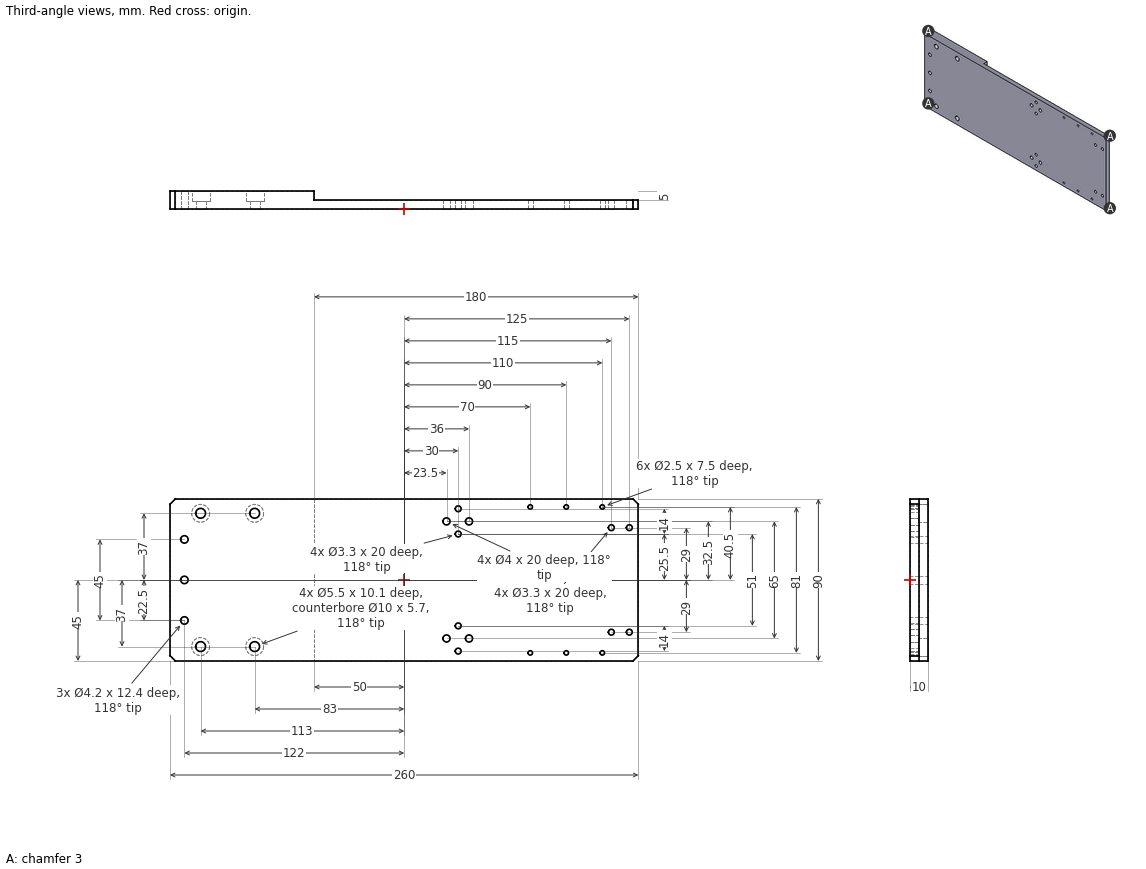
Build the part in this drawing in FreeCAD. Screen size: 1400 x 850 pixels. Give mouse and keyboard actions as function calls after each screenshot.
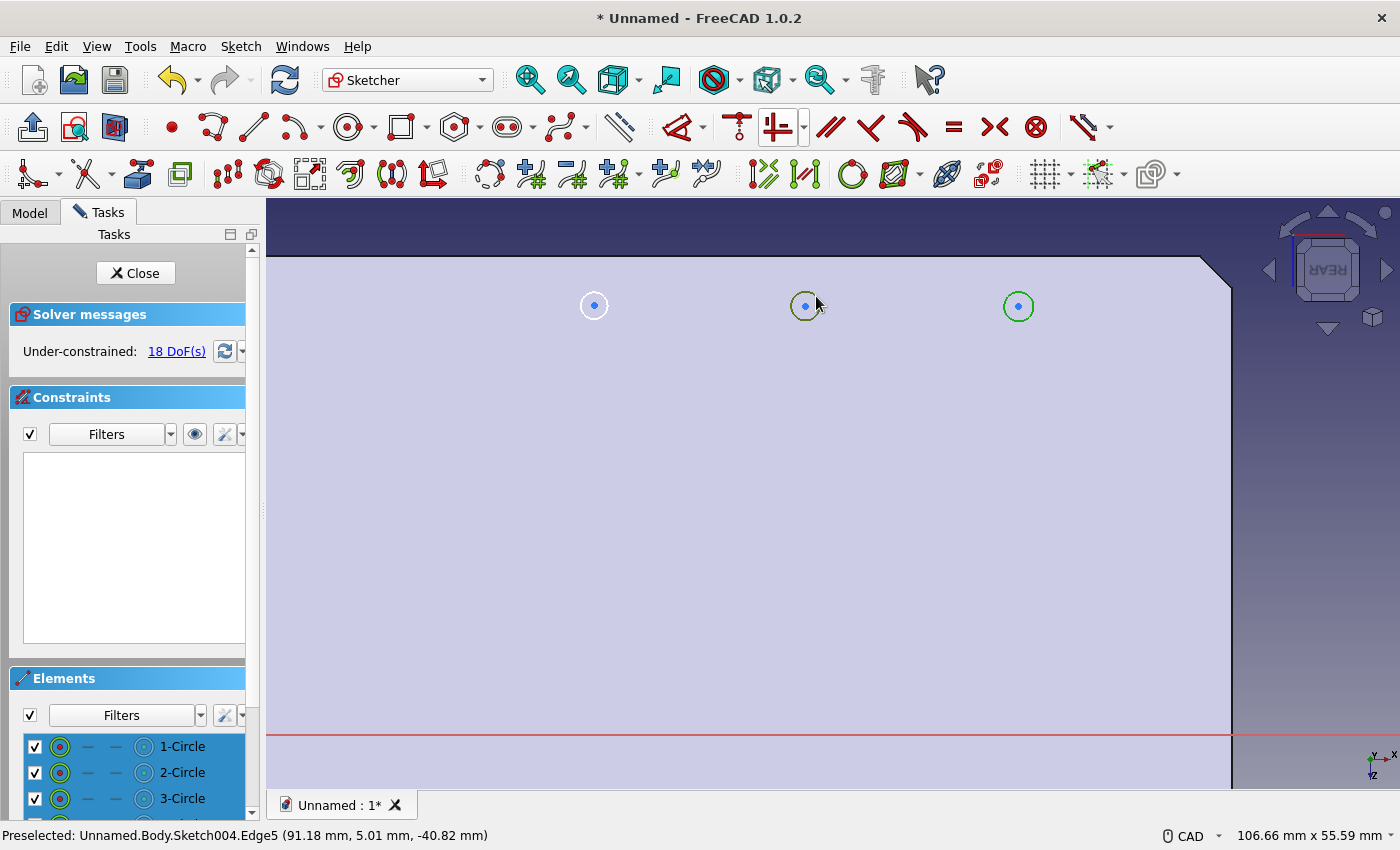
click(604, 296)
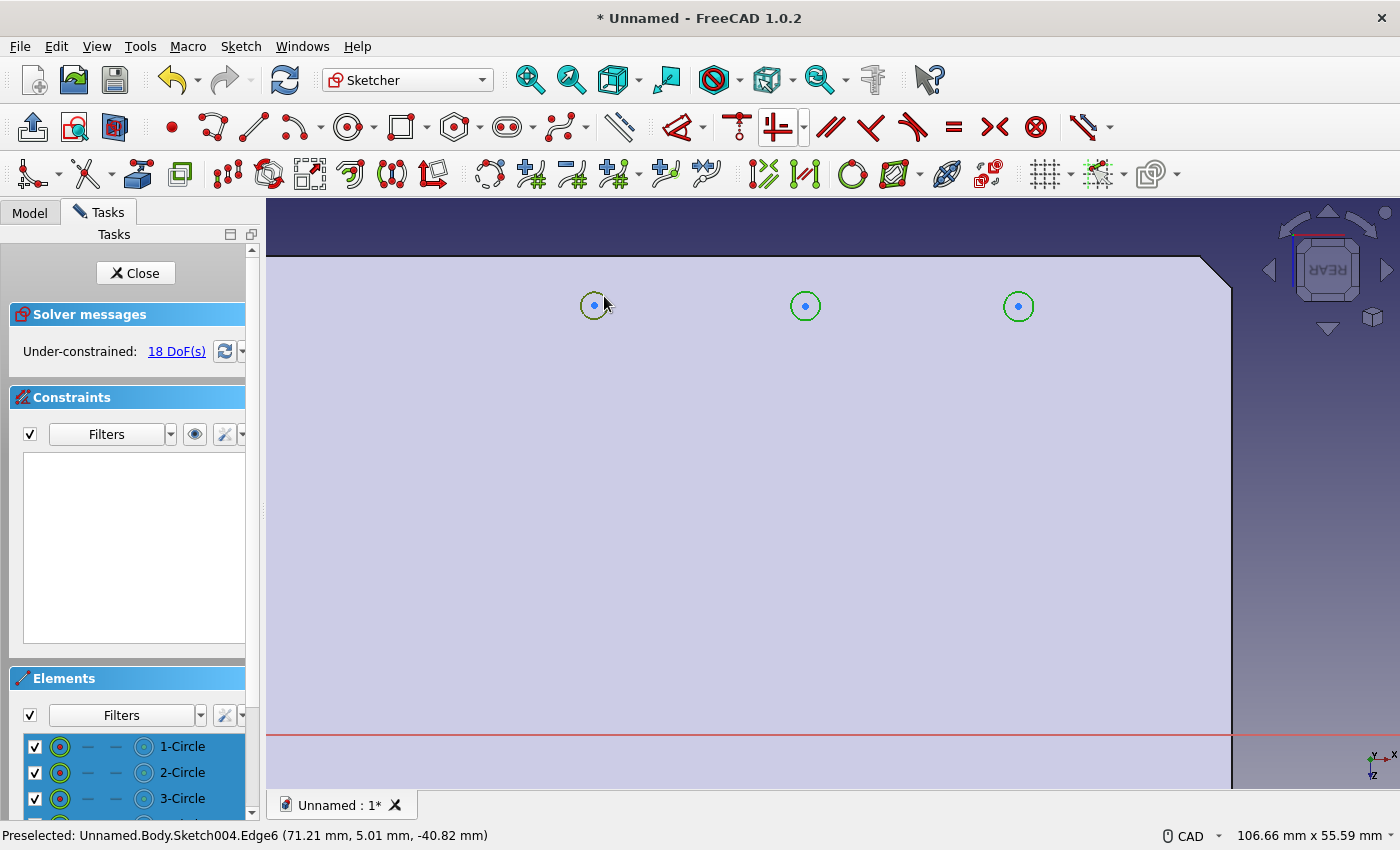
click(954, 128)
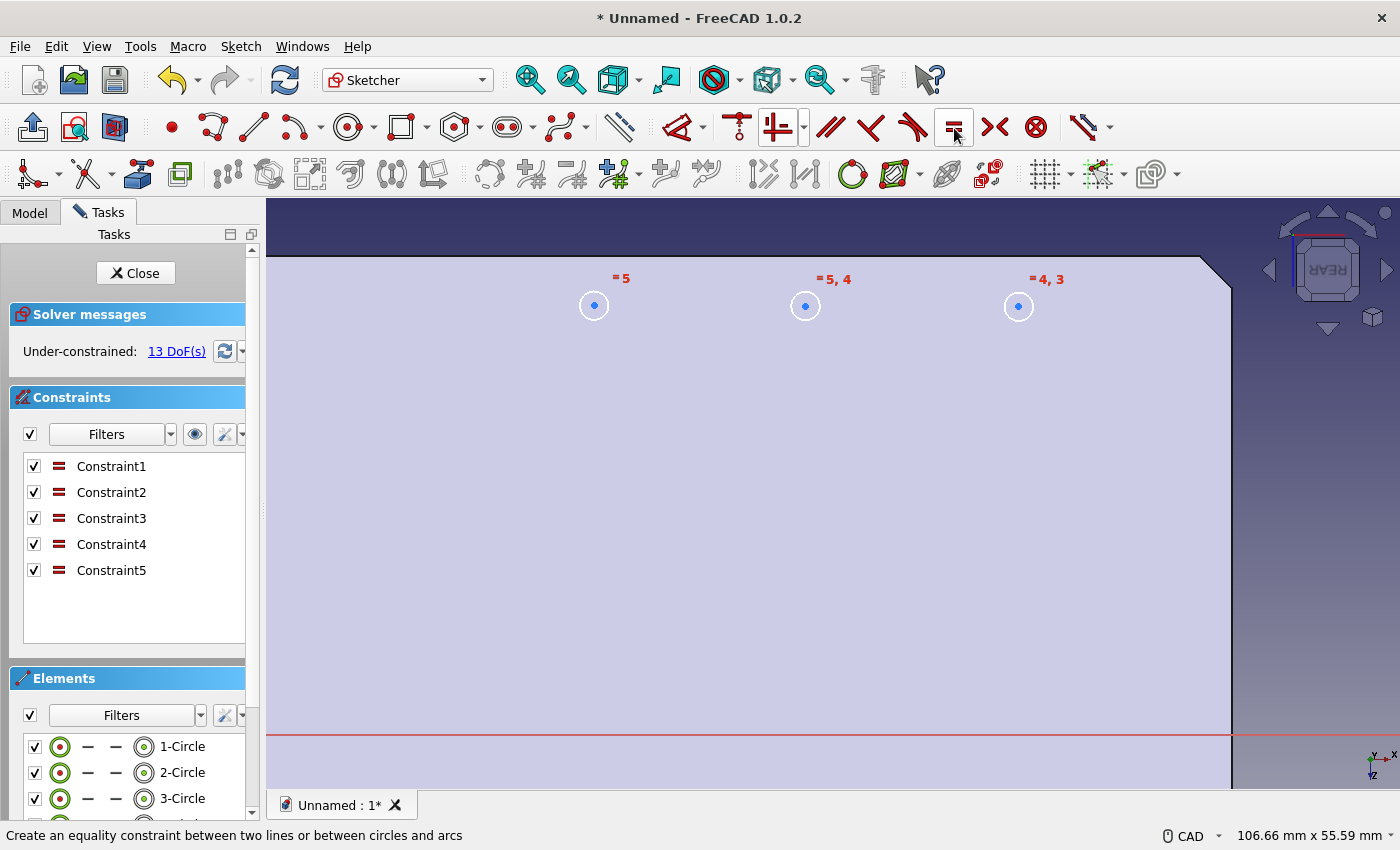
scroll(1029, 297, down, 4)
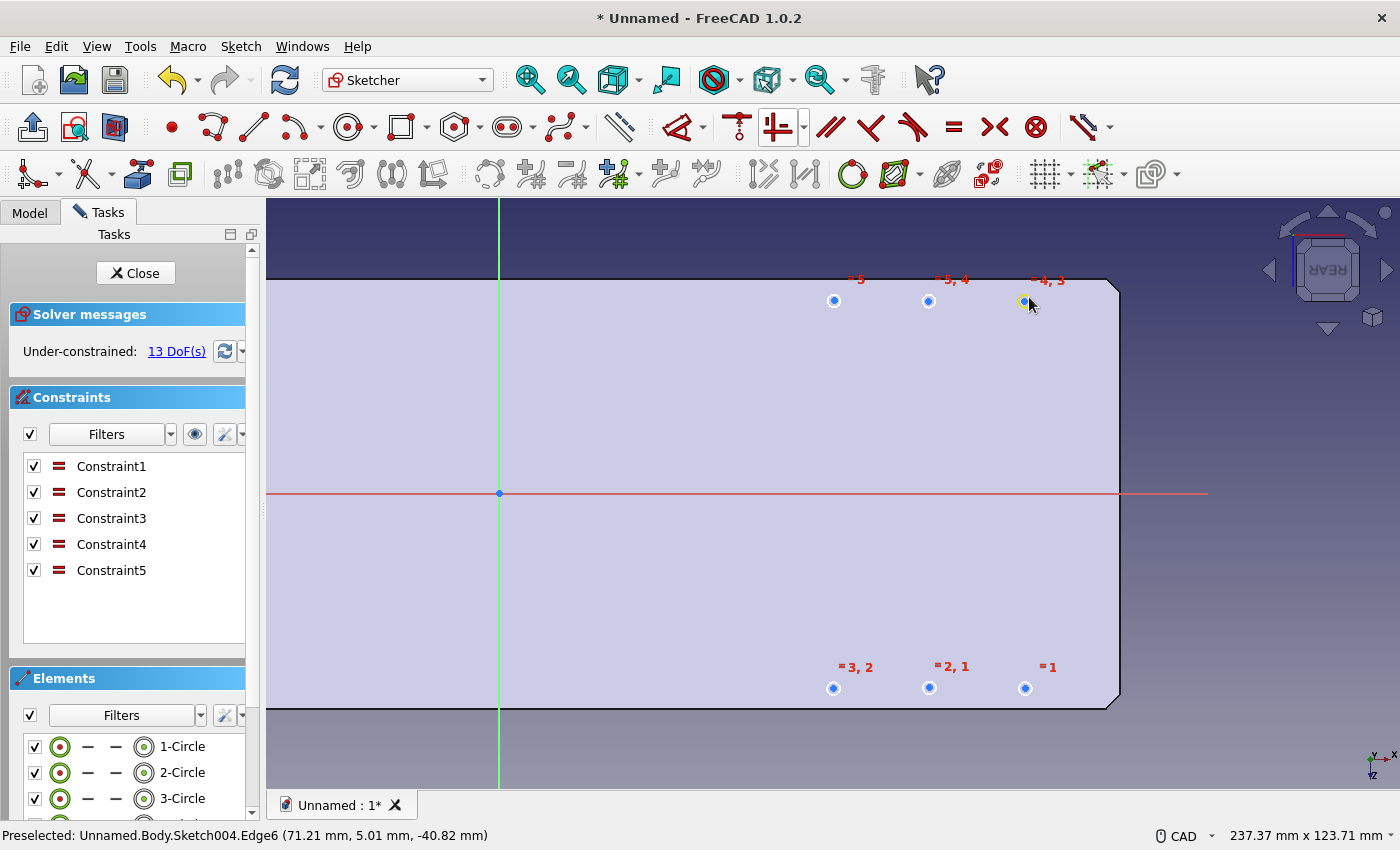
click(1025, 689)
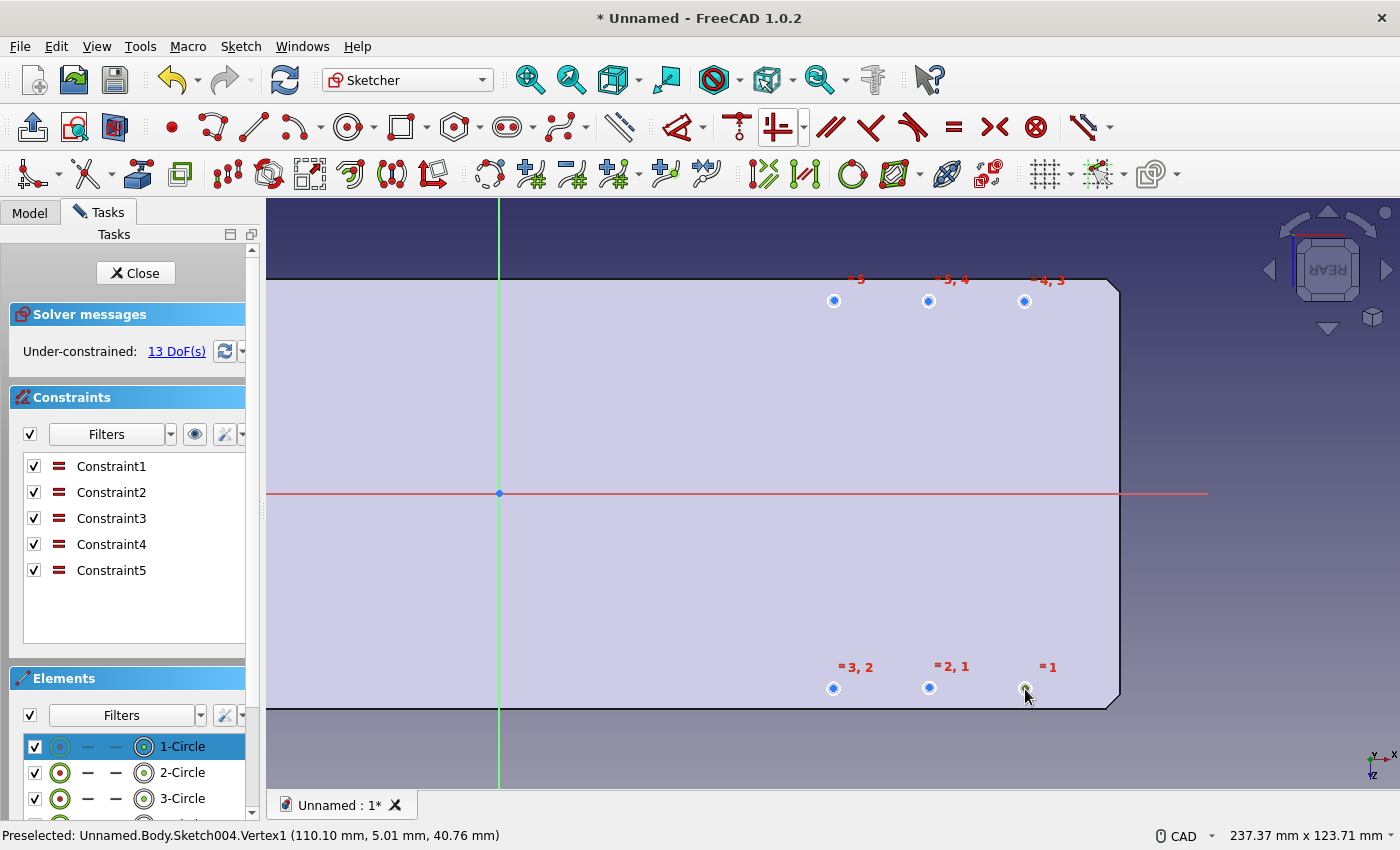
click(929, 688)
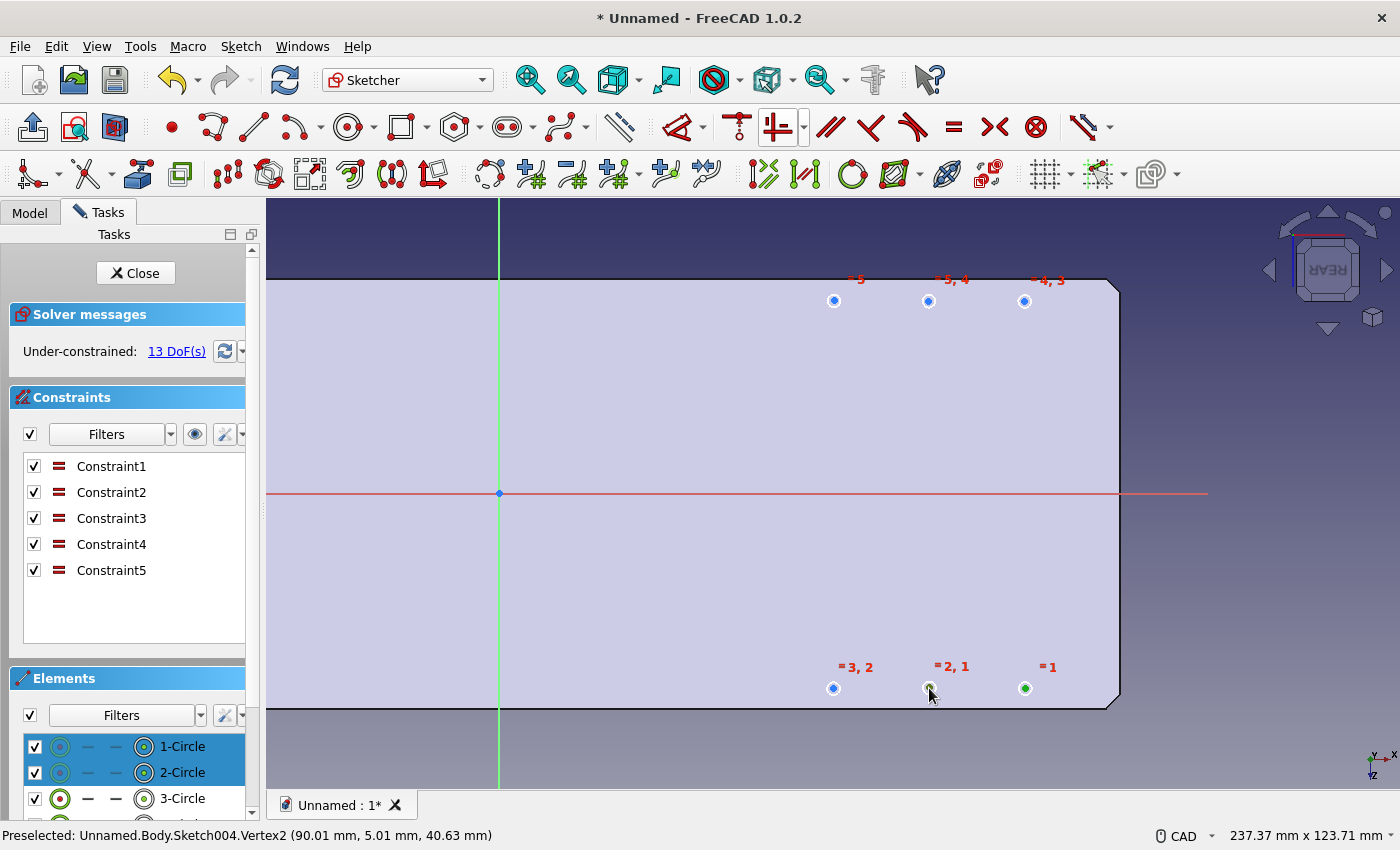
click(804, 128)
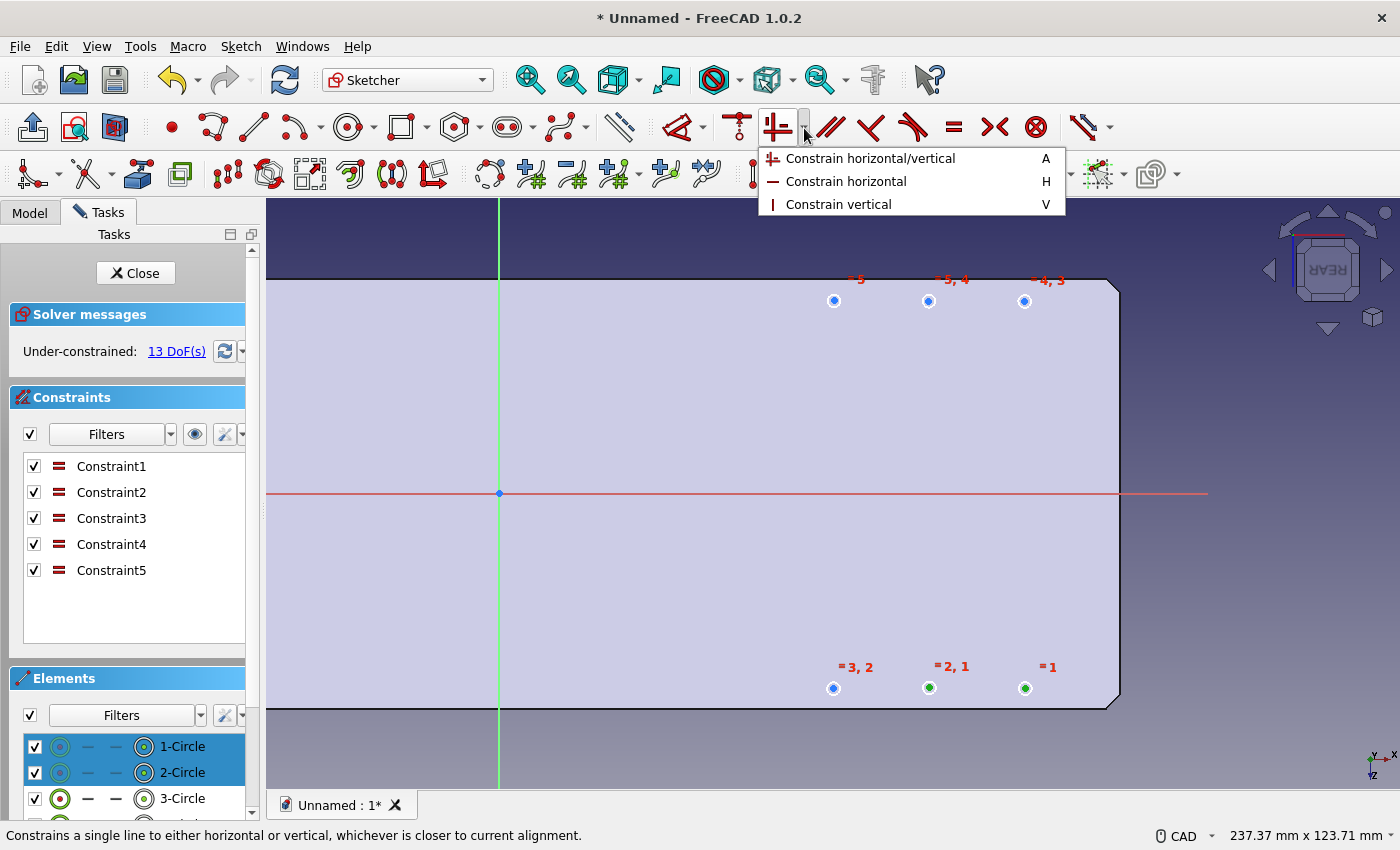
click(912, 182)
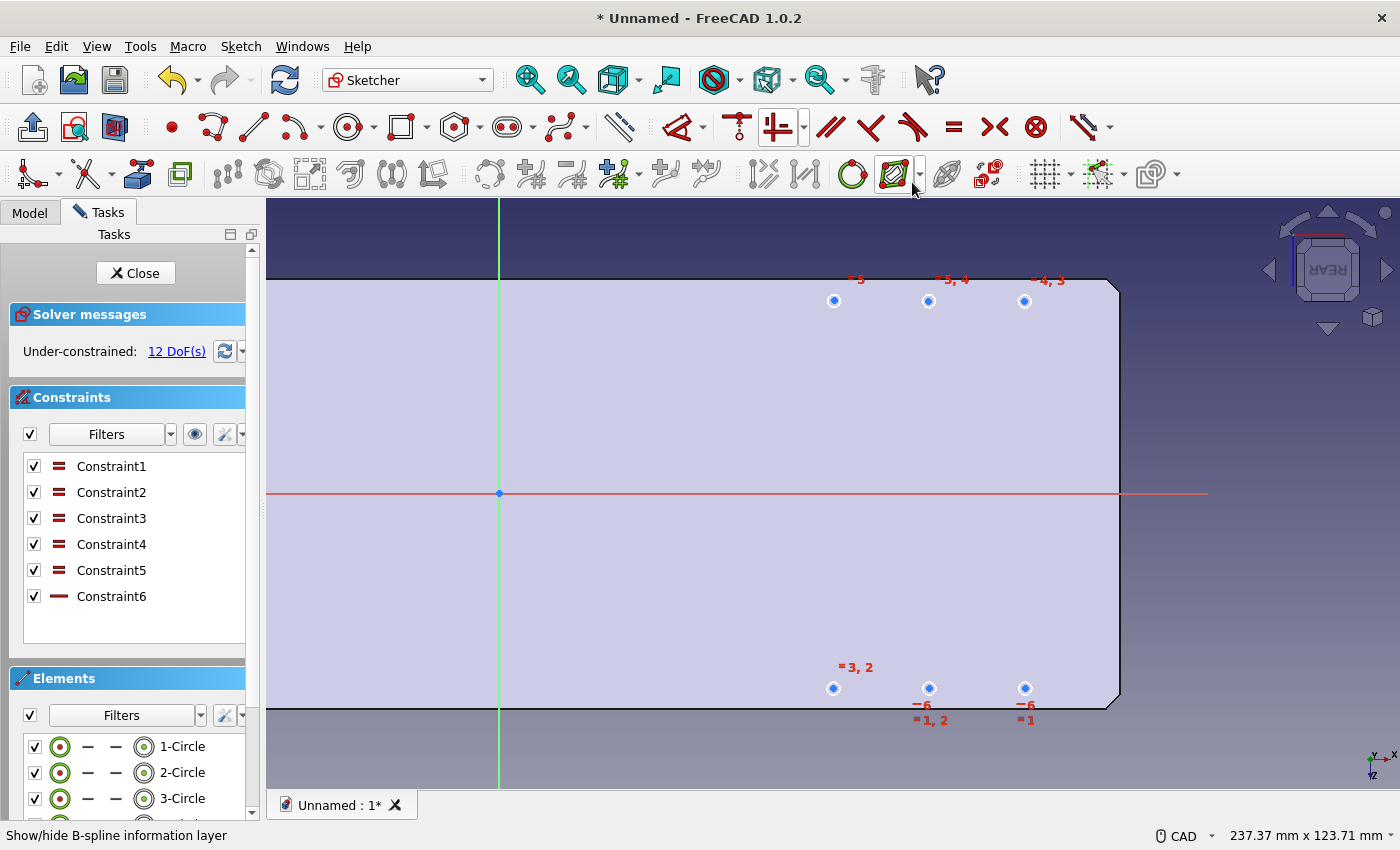
click(929, 689)